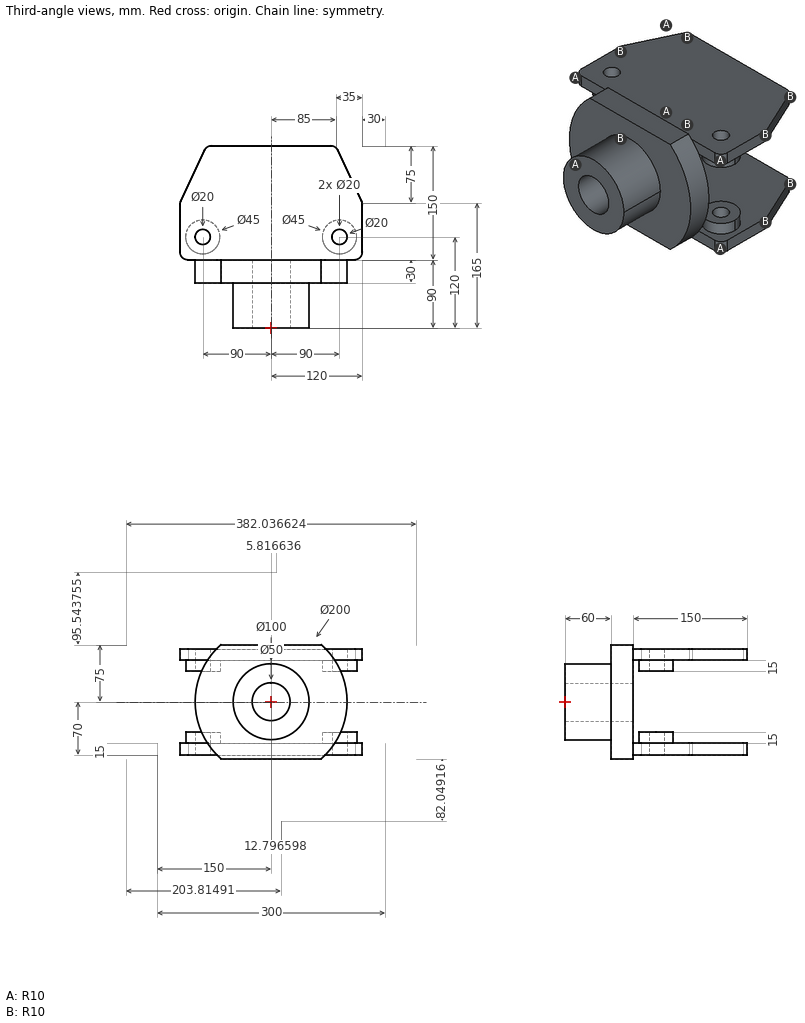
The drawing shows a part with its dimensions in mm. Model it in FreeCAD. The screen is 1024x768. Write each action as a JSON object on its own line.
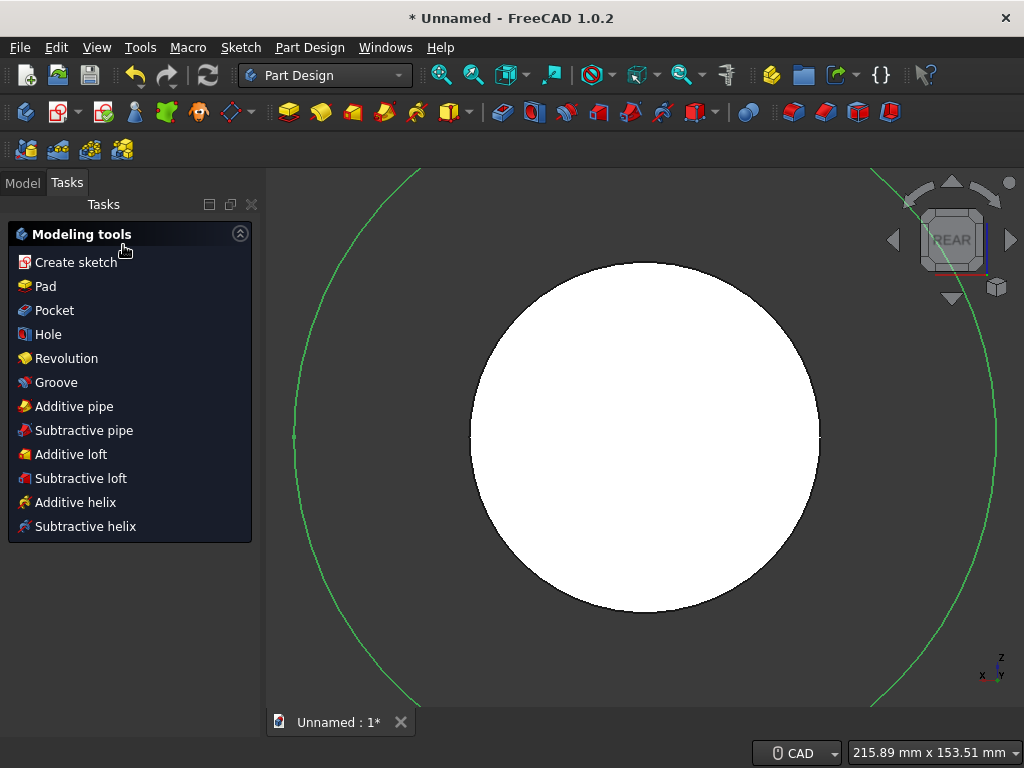
{"action": "left_click", "coordinate": [290, 112]}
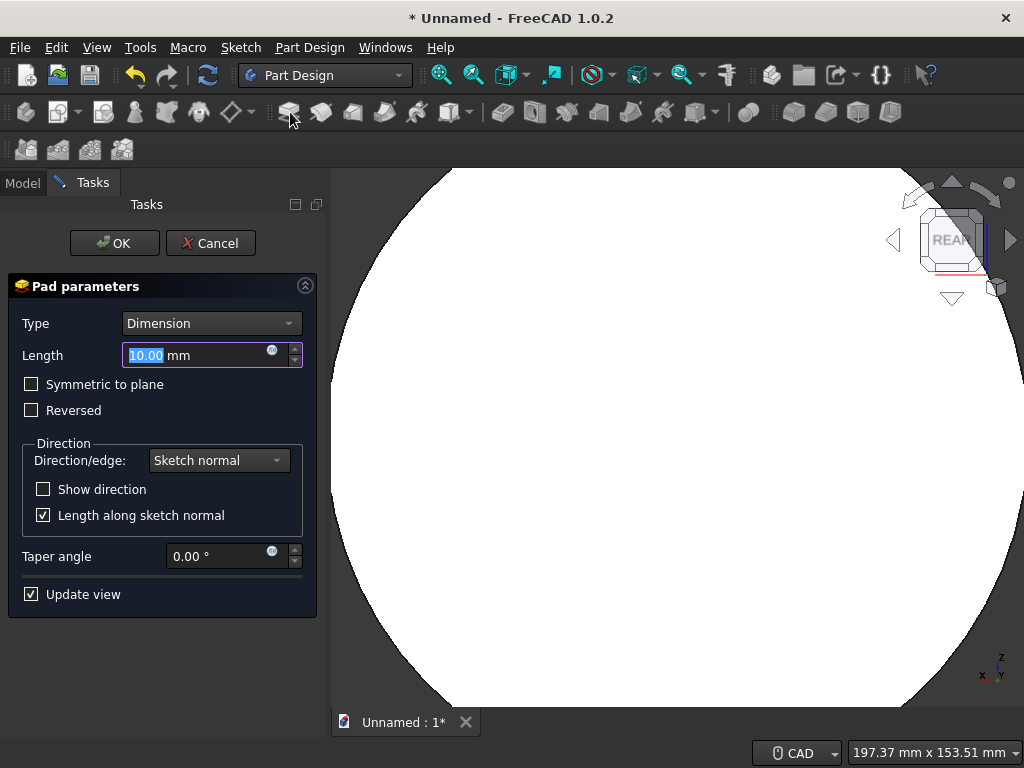
{"action": "type", "text": "30"}
{"action": "key", "text": "Tab"}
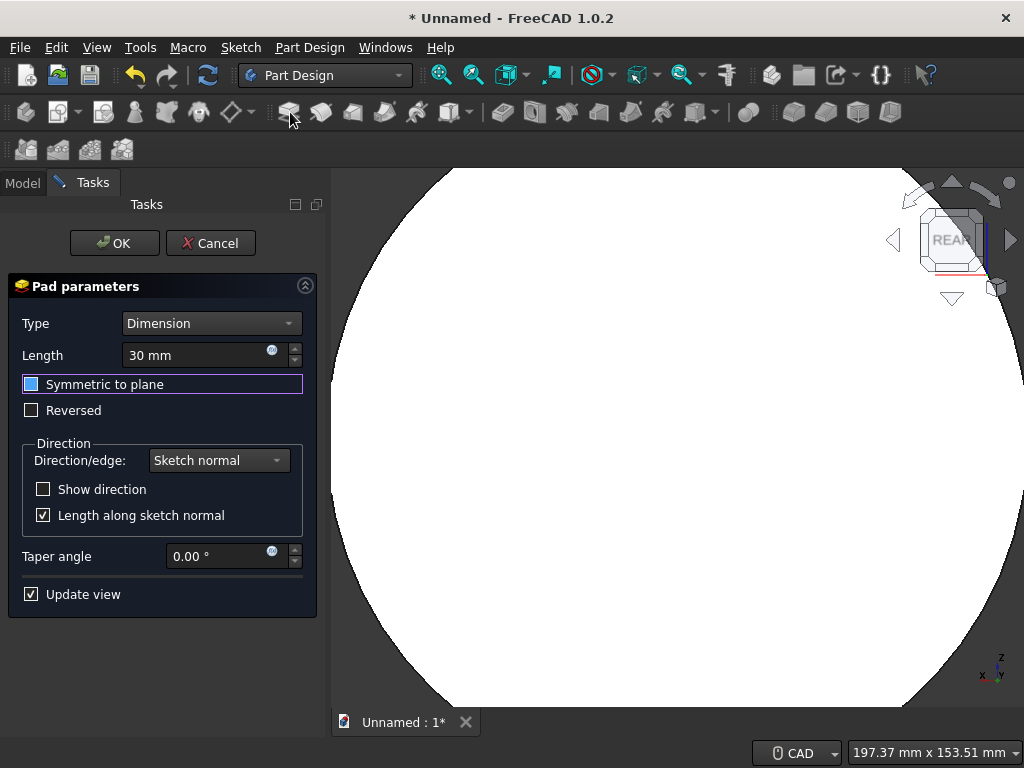
{"action": "left_click", "coordinate": [115, 243]}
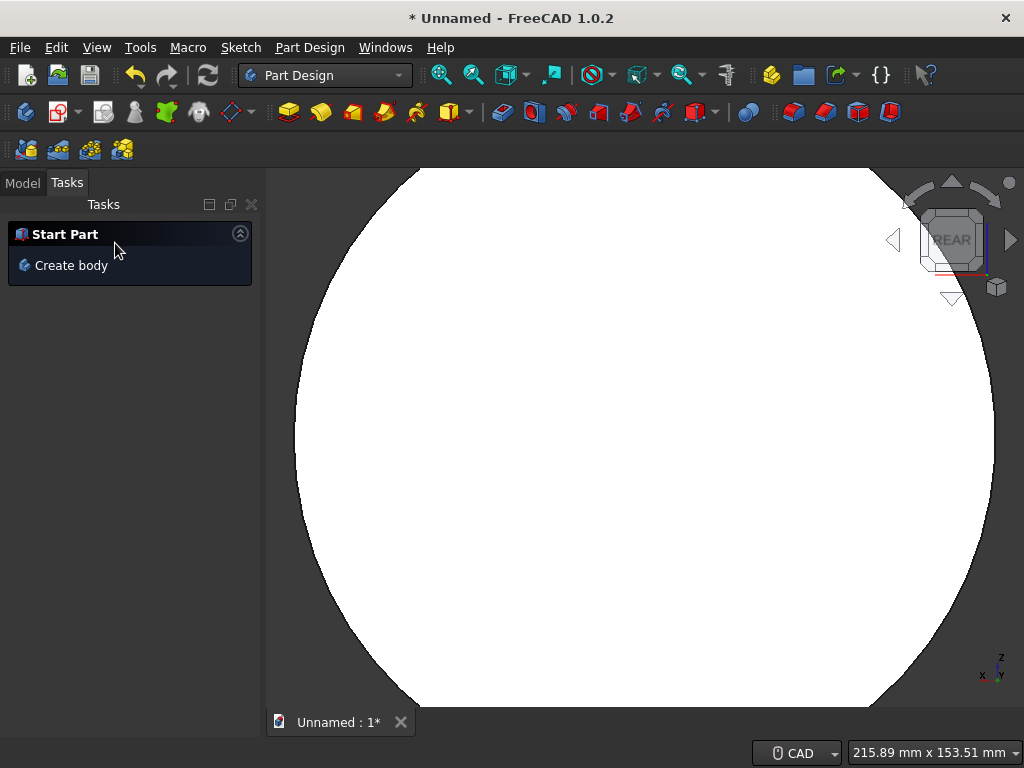
{"action": "left_click", "coordinate": [442, 76]}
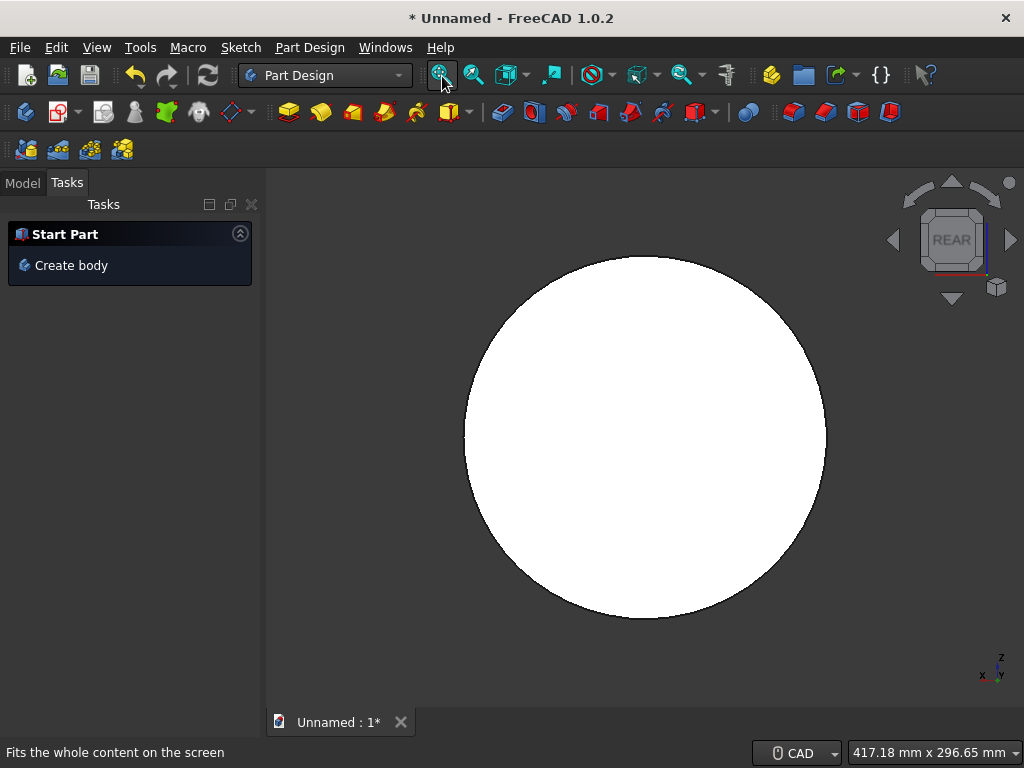
{"action": "key", "text": "0"}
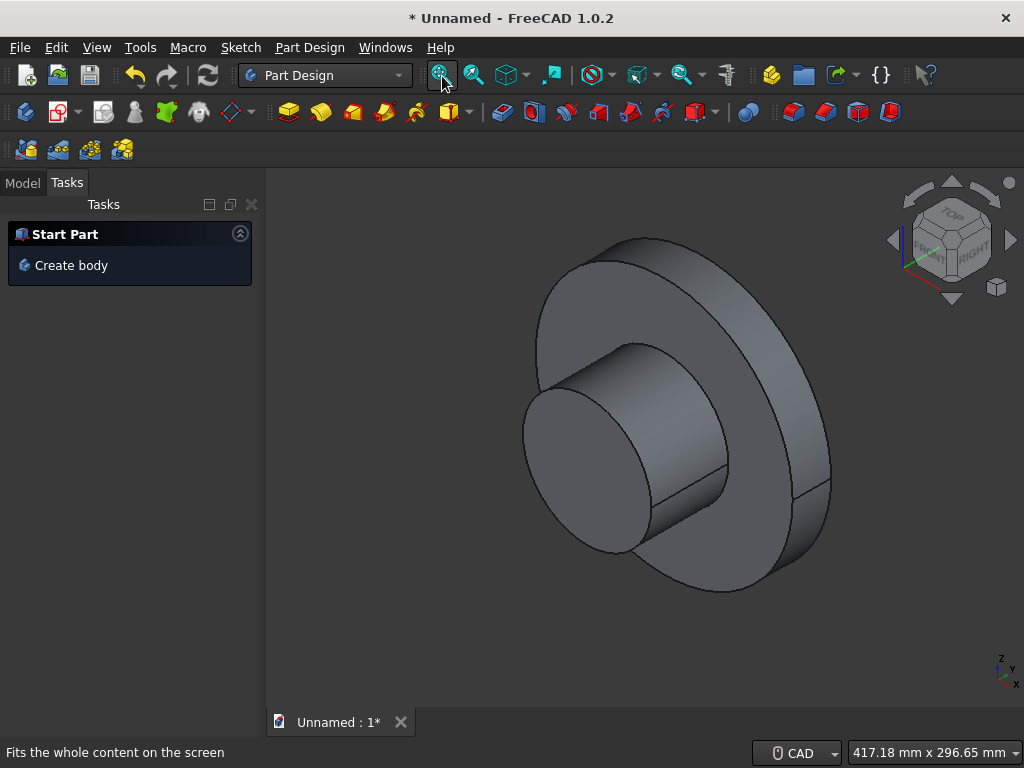
{"action": "left_click", "coordinate": [738, 552]}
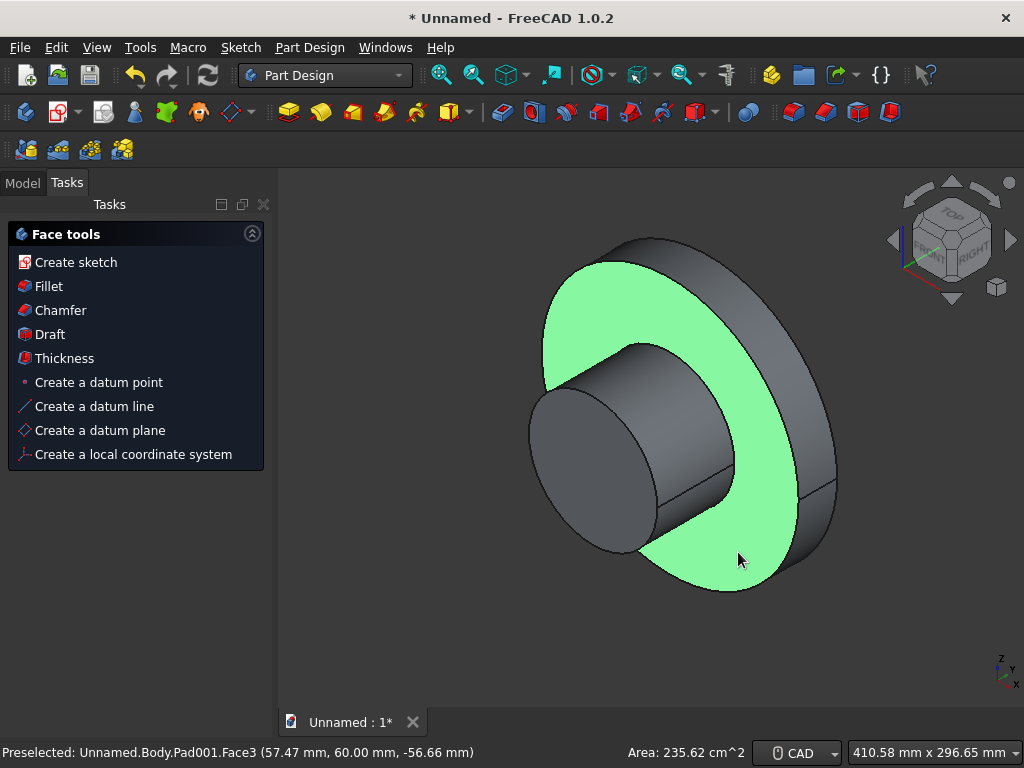
{"action": "left_click", "coordinate": [58, 112]}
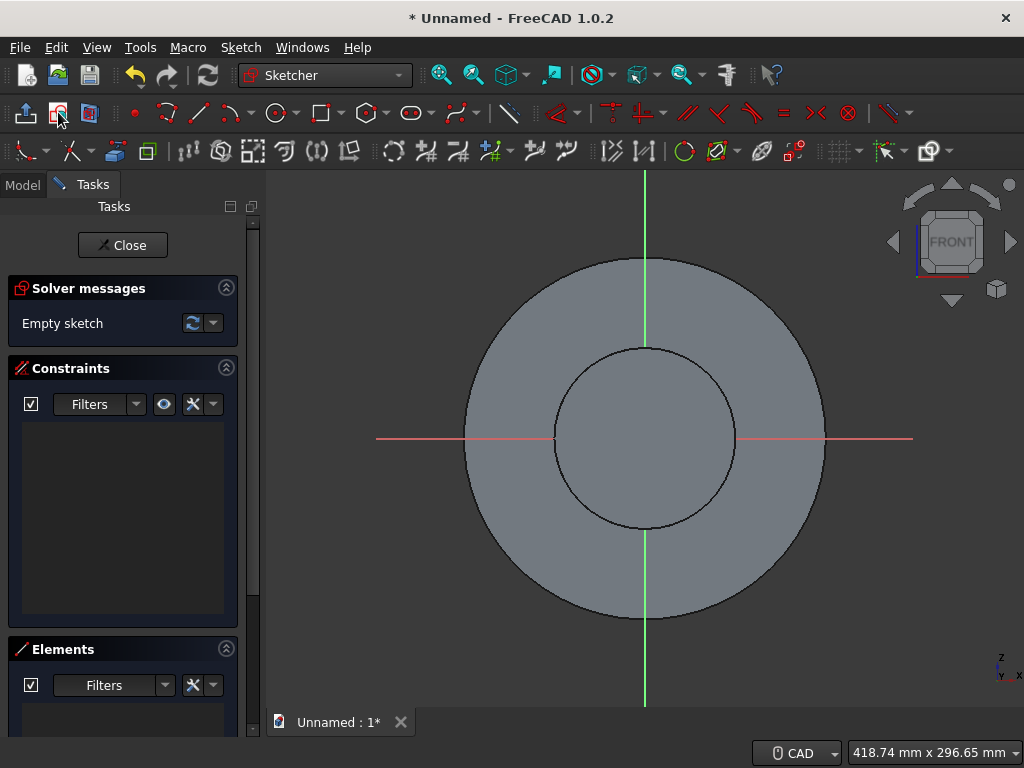
{"action": "scroll", "coordinate": [493, 453], "scroll_direction": "down", "scroll_amount": 3}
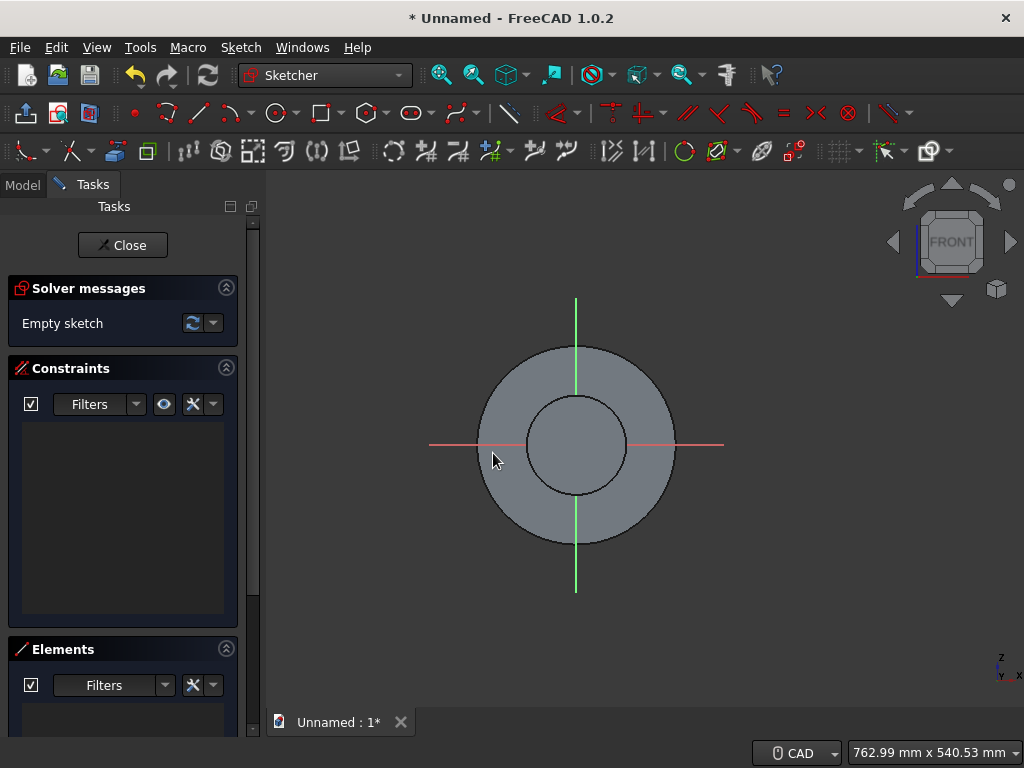
{"action": "left_click", "coordinate": [168, 114]}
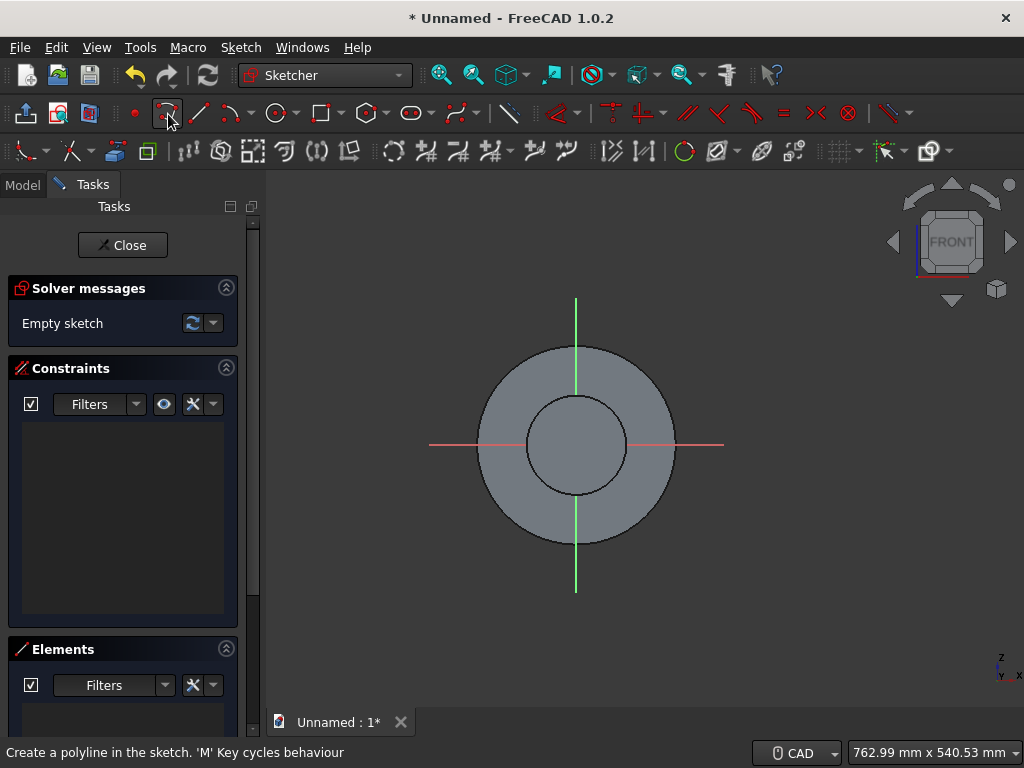
{"action": "scroll", "coordinate": [582, 276], "scroll_direction": "up", "scroll_amount": 6}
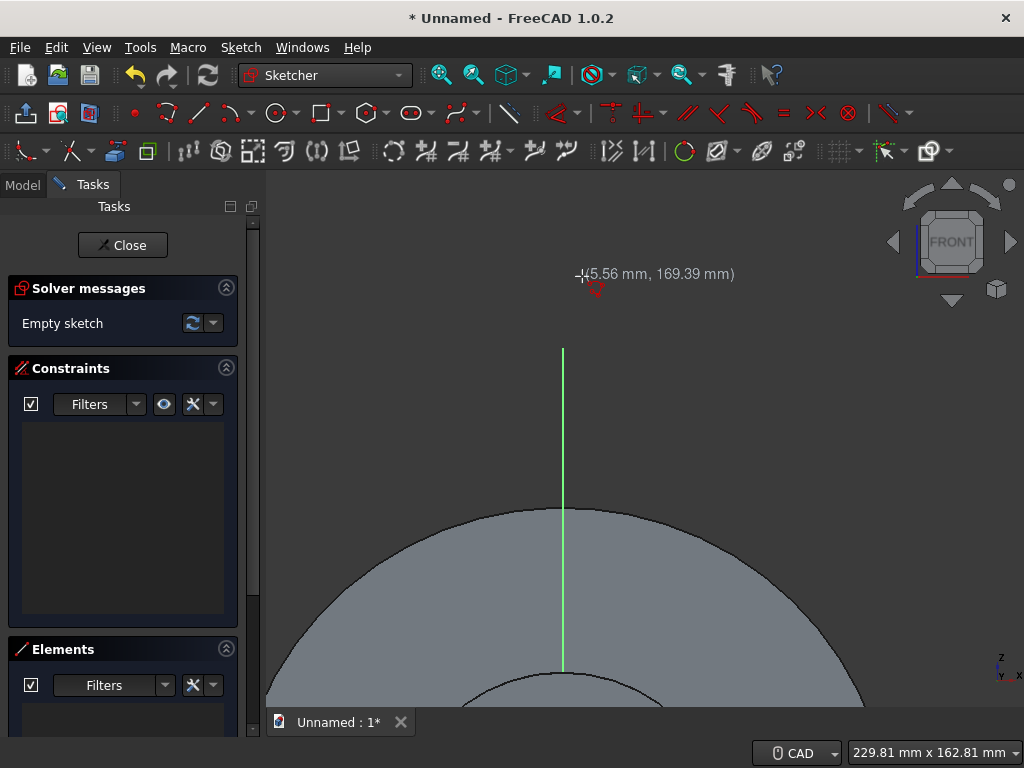
{"action": "left_click", "coordinate": [582, 275]}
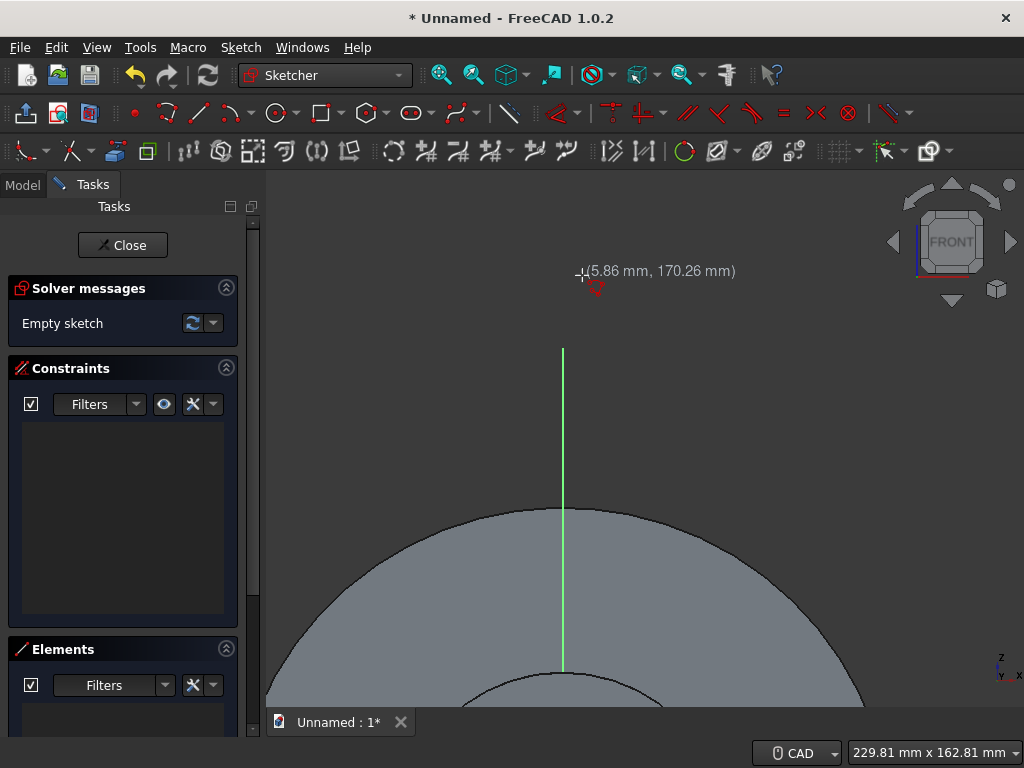
{"action": "scroll", "coordinate": [582, 276], "scroll_direction": "down", "scroll_amount": 6}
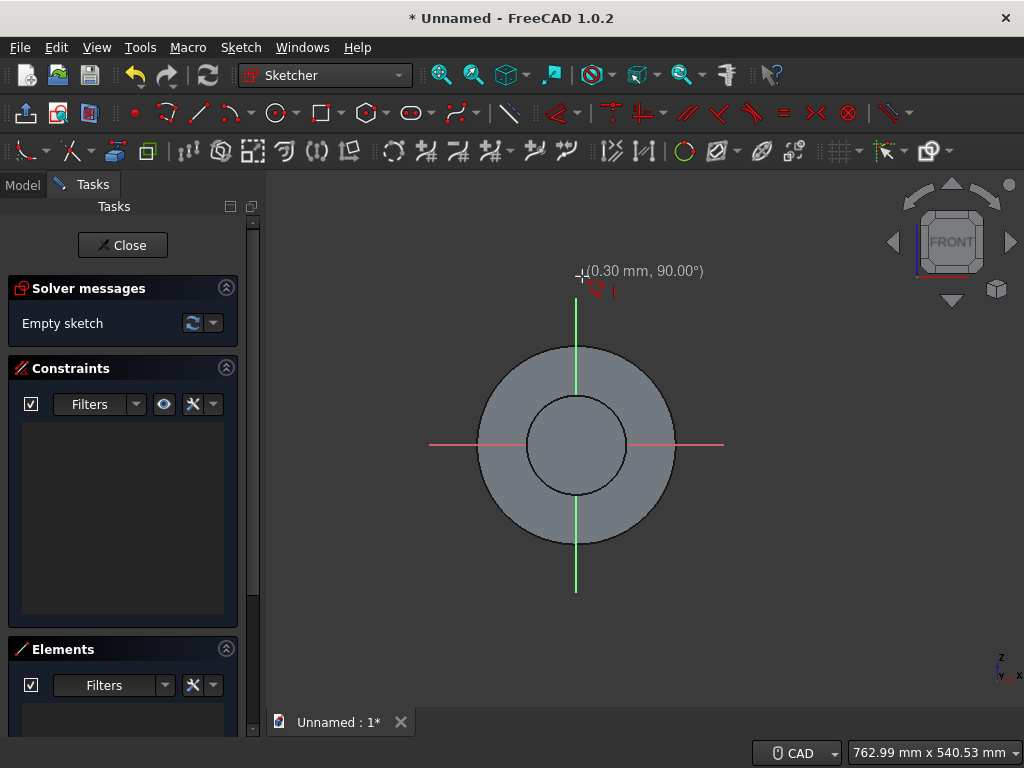
{"action": "left_click", "coordinate": [387, 371]}
{"action": "left_click", "coordinate": [766, 371]}